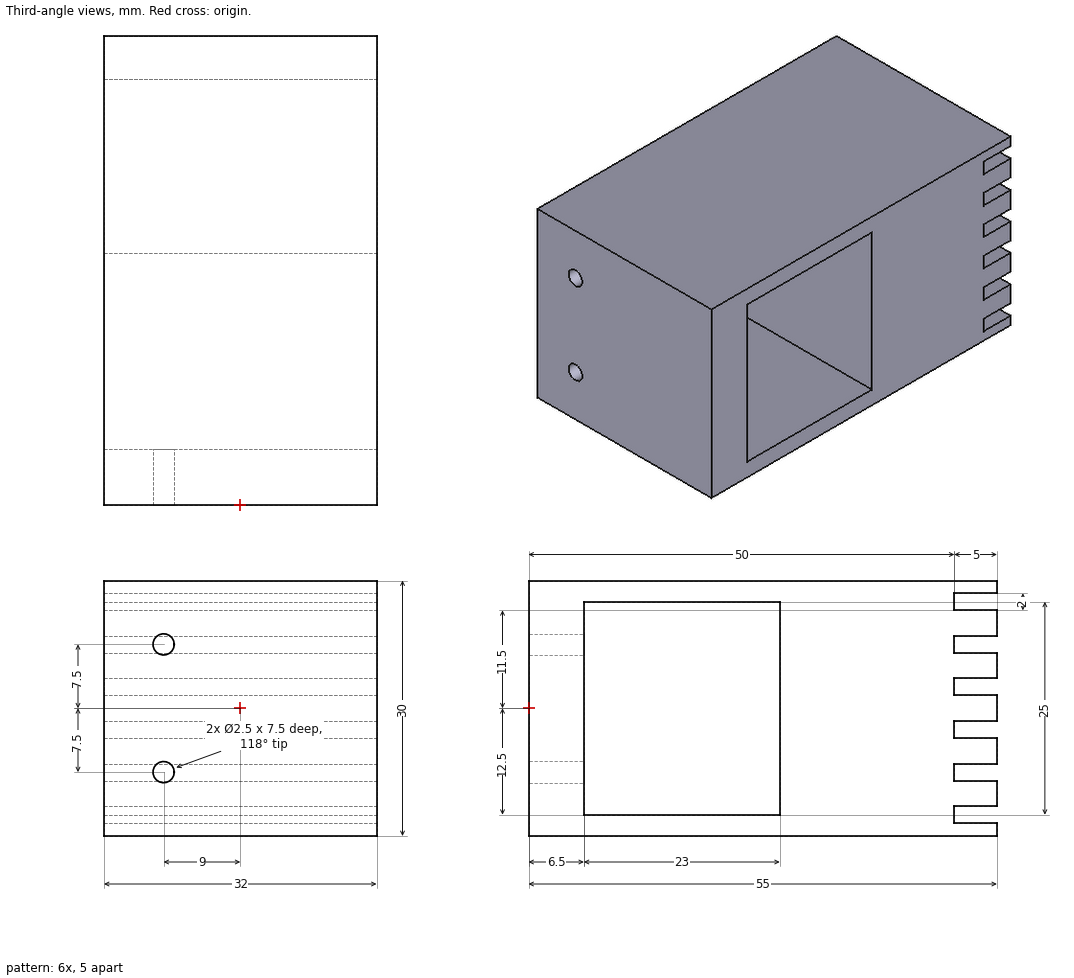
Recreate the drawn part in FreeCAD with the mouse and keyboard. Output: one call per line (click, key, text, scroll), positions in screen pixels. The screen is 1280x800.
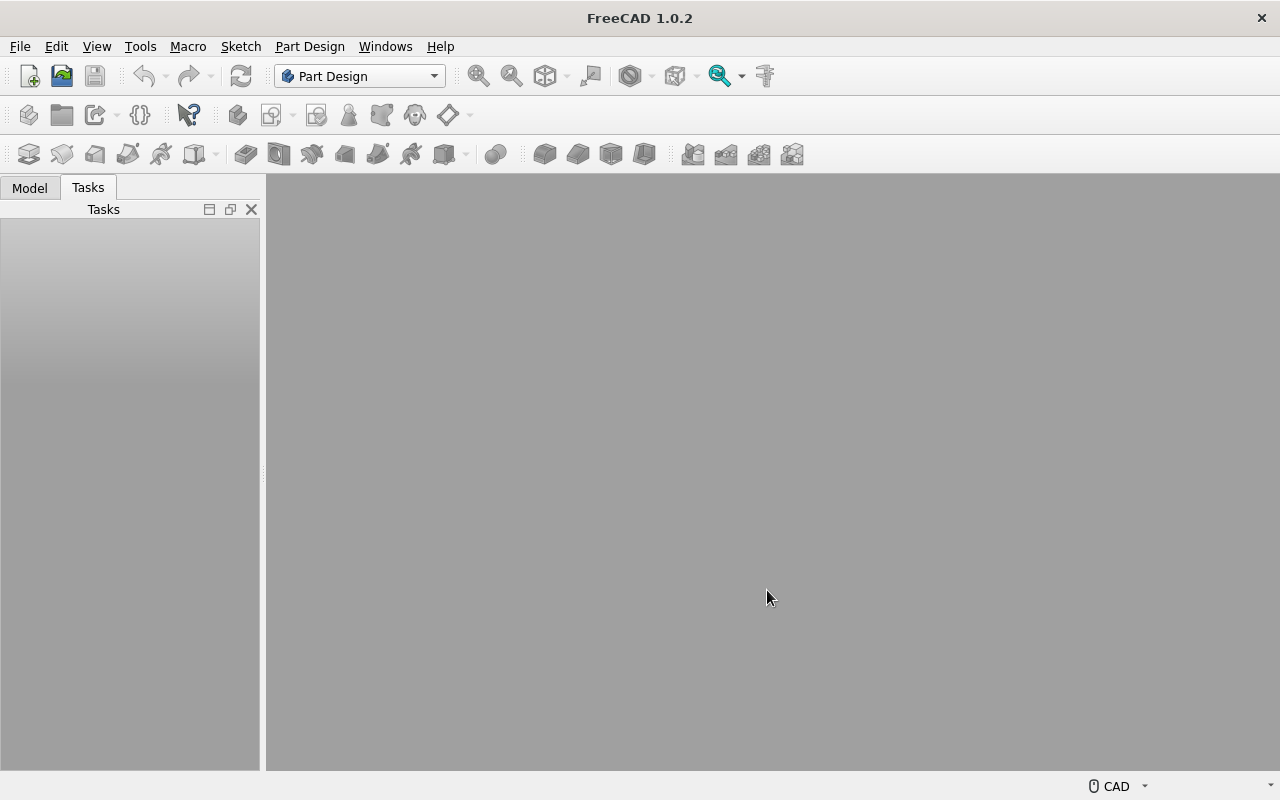
click(29, 76)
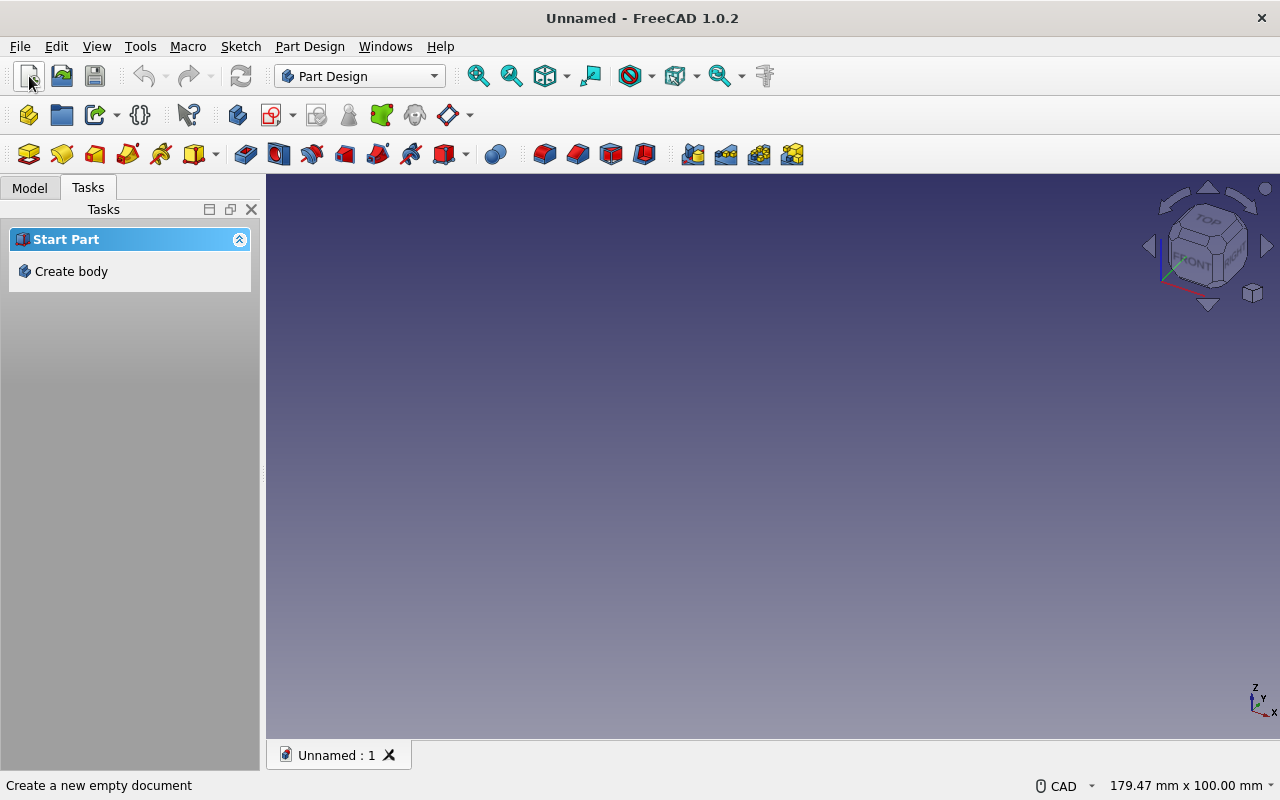
click(270, 116)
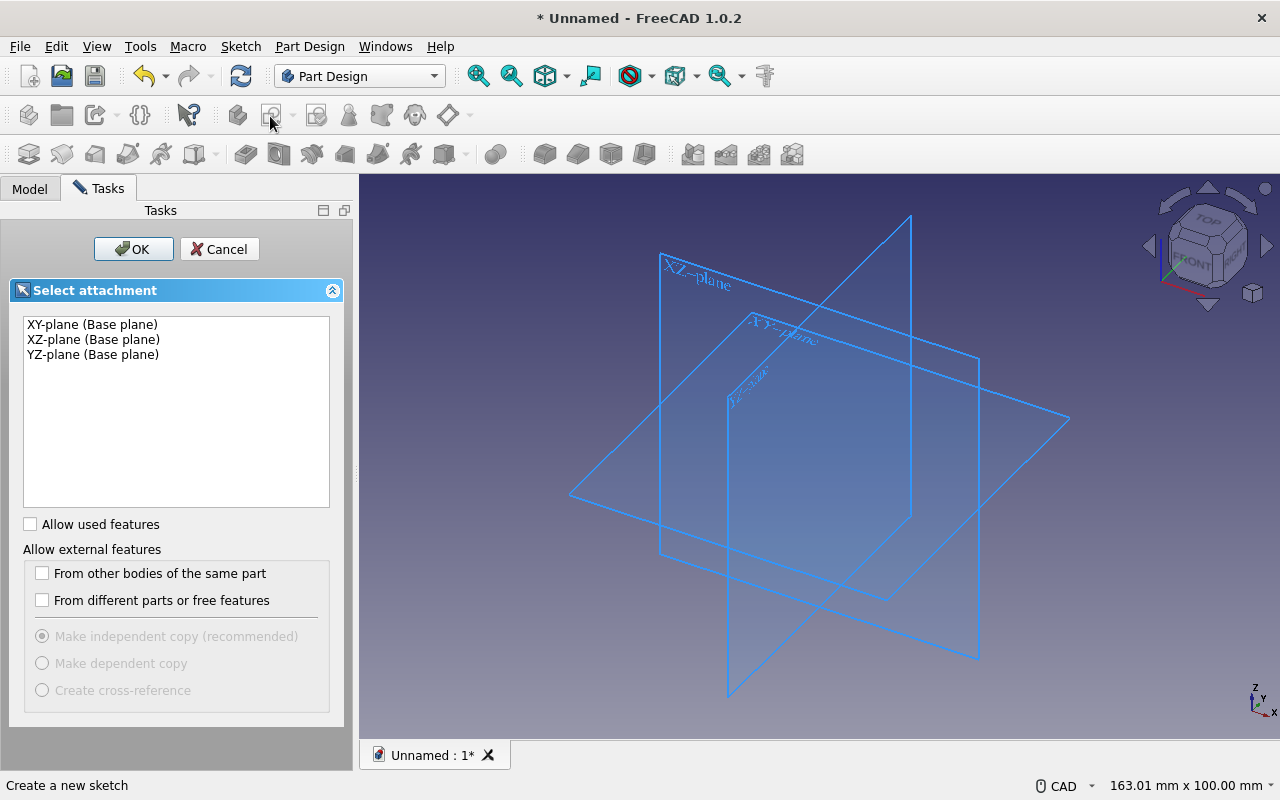
click(84, 340)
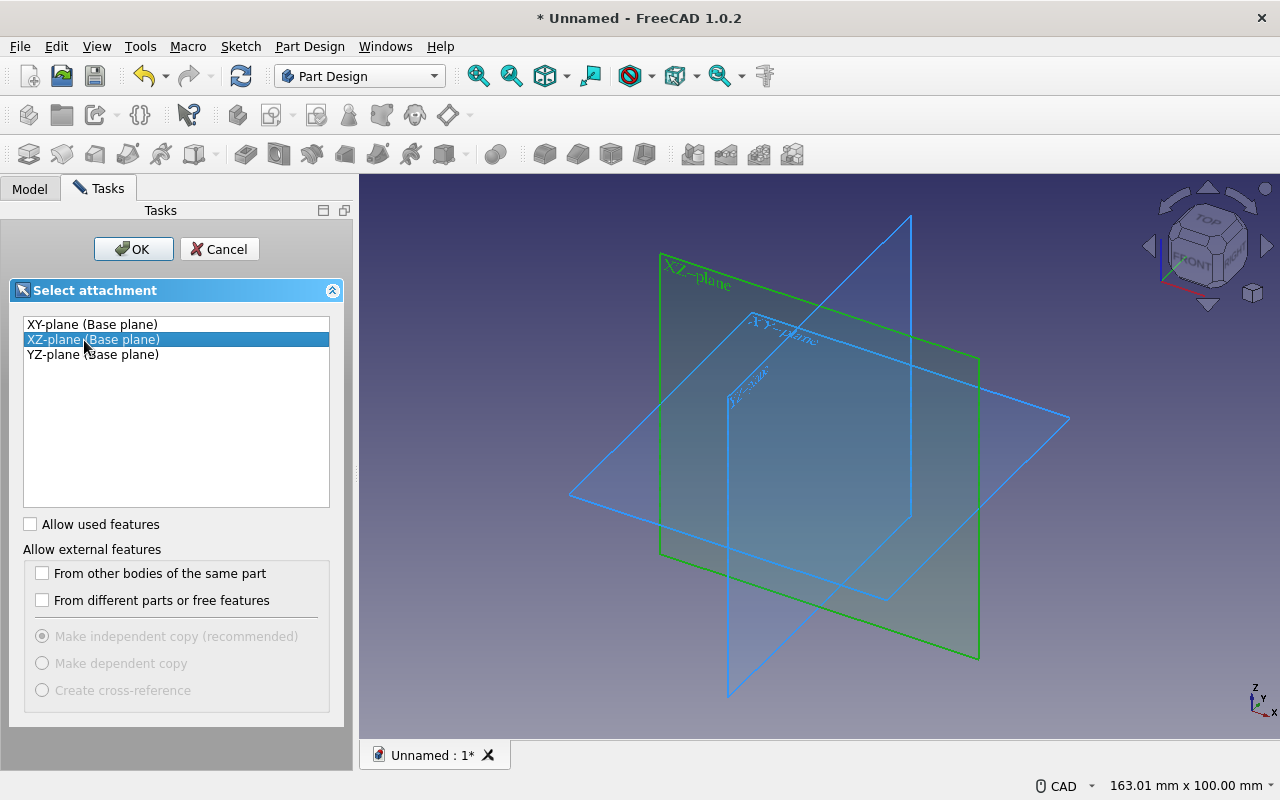
click(134, 249)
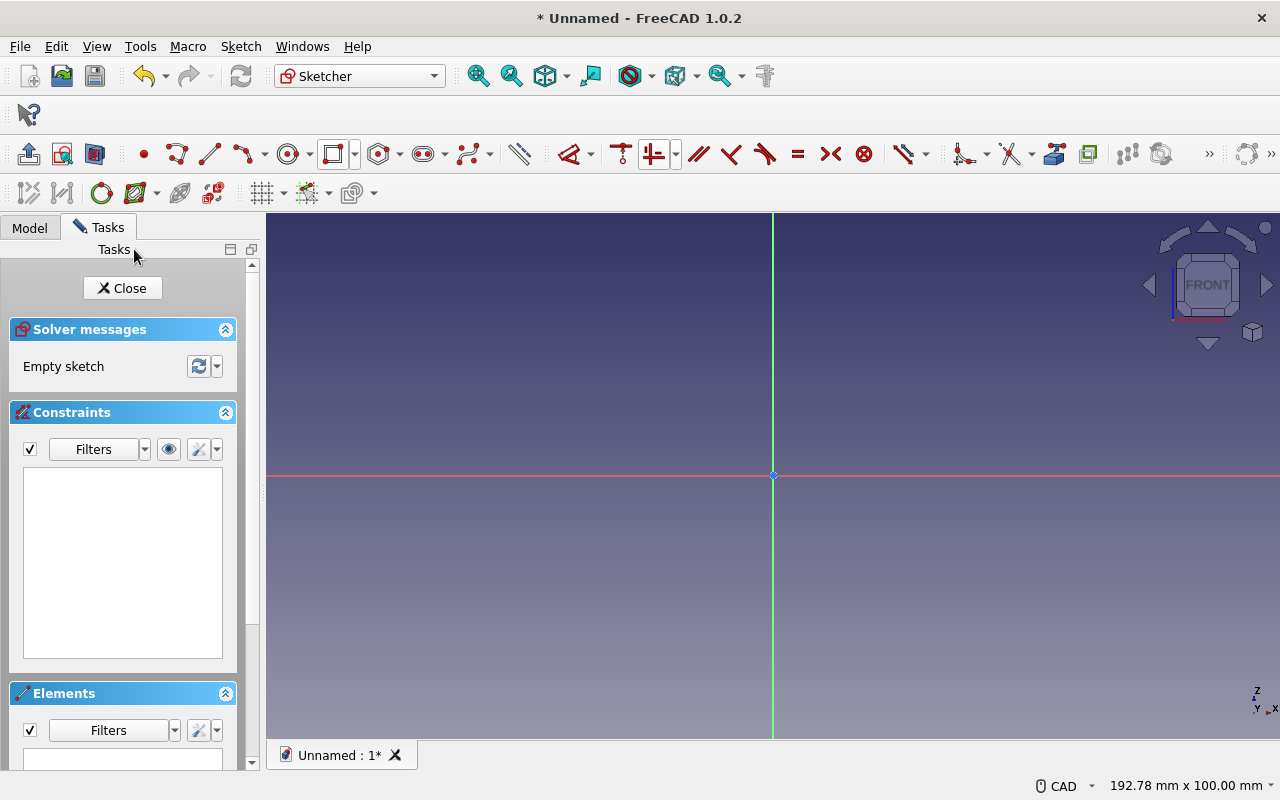
scroll(829, 476, up, 4)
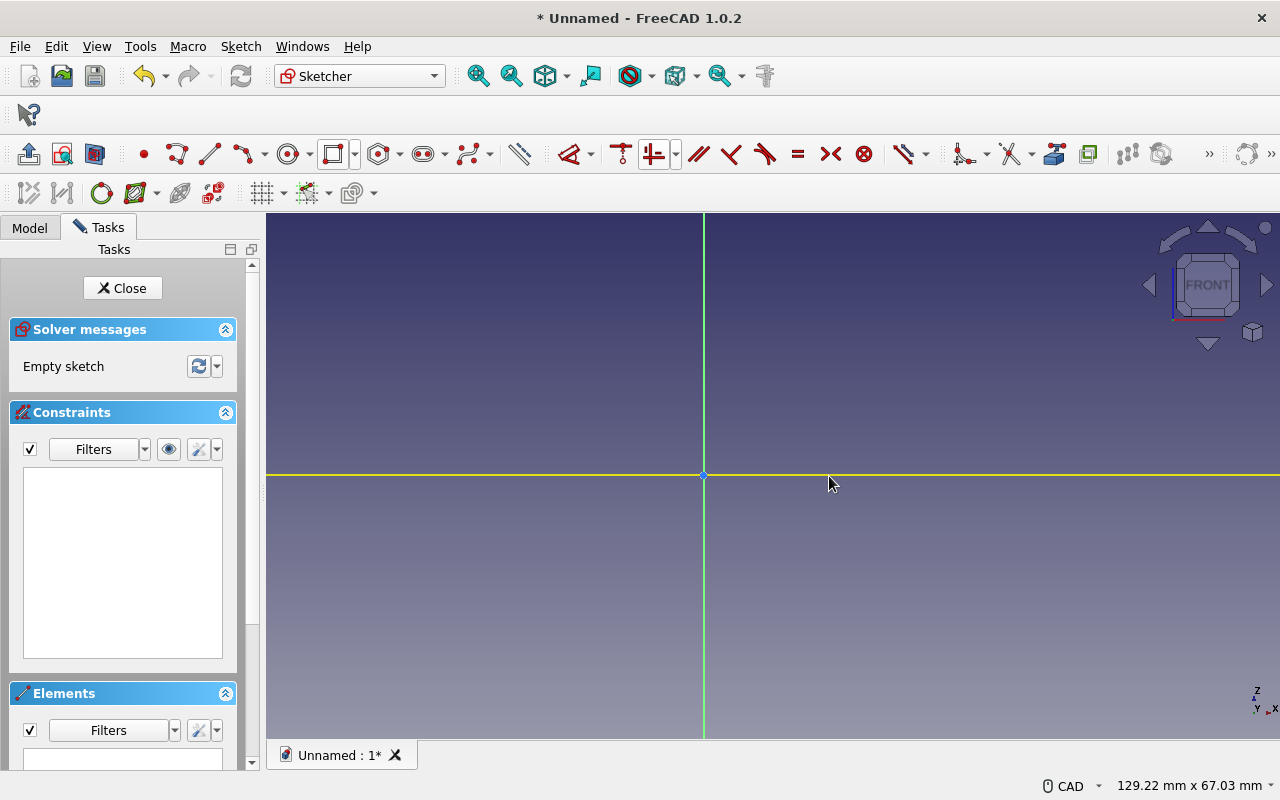
click(354, 154)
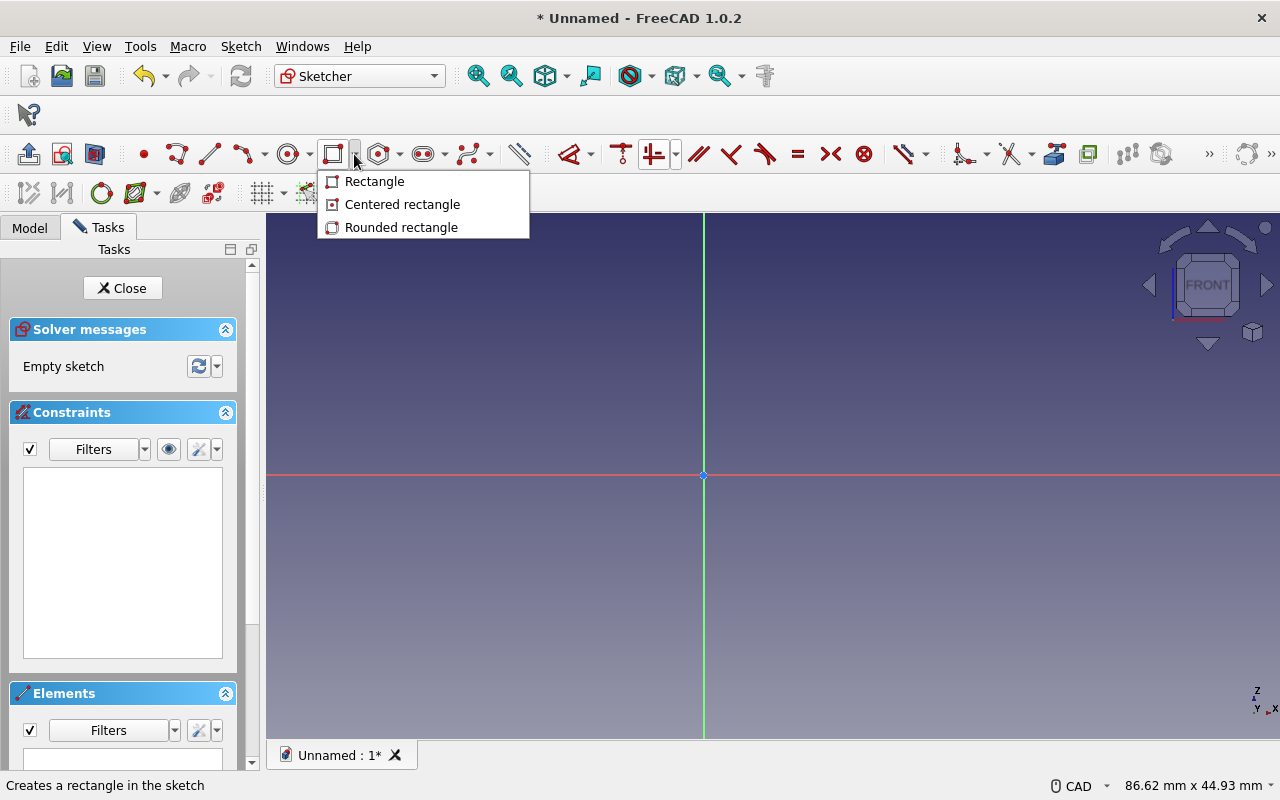
click(424, 204)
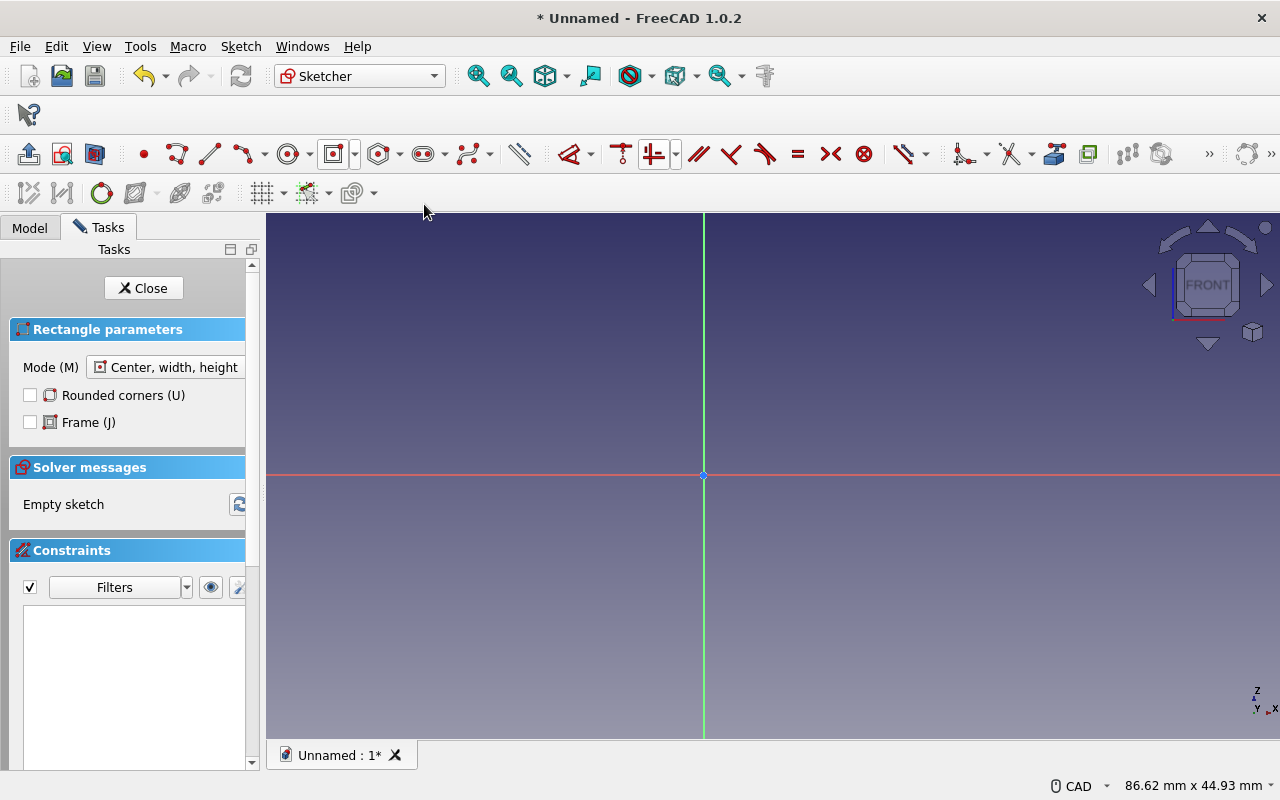
click(704, 475)
click(891, 300)
key(Escape)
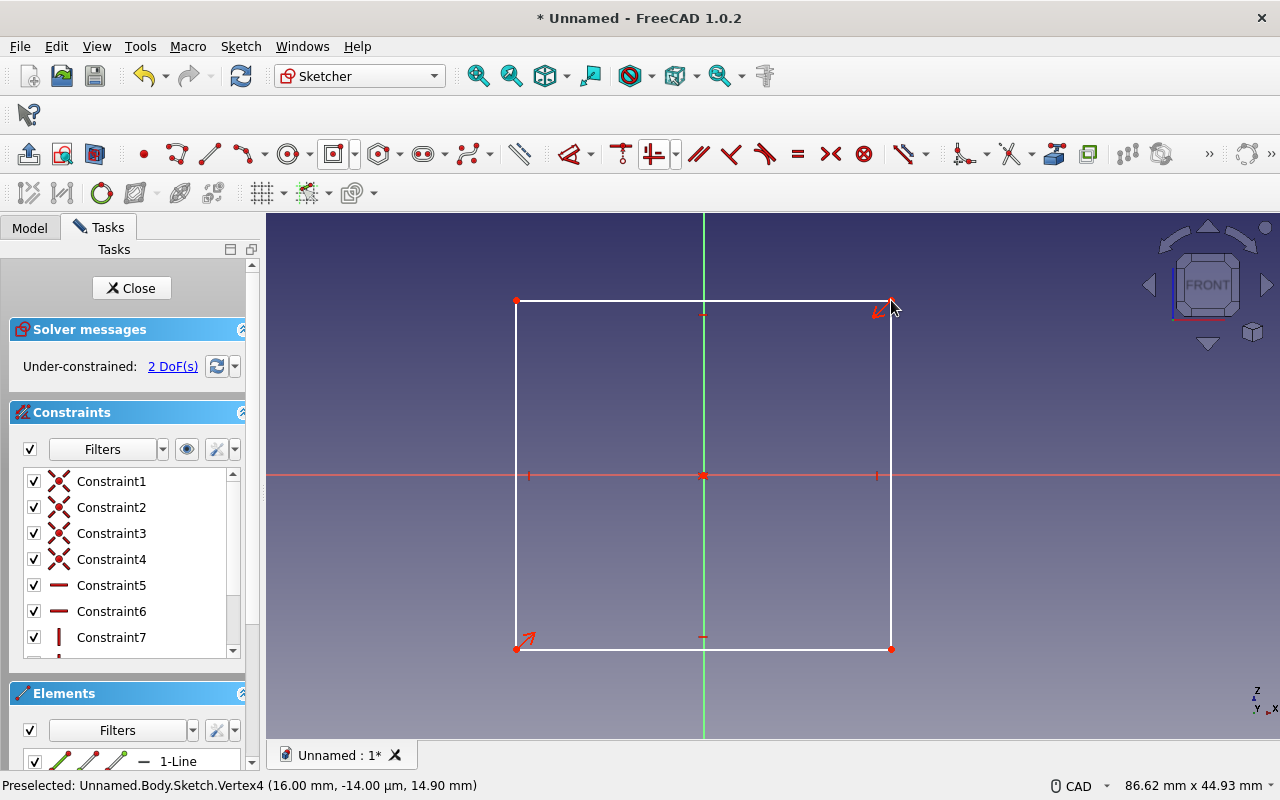
click(568, 154)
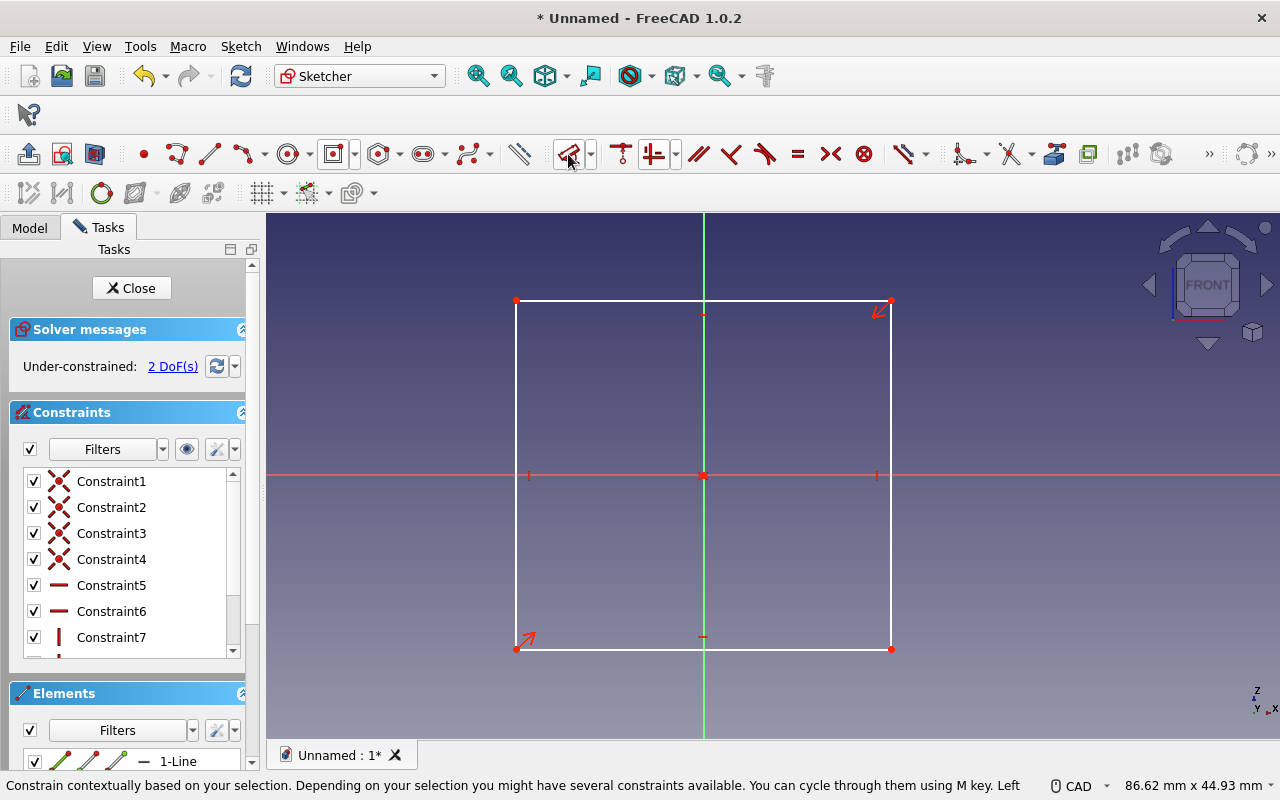
click(629, 650)
click(618, 684)